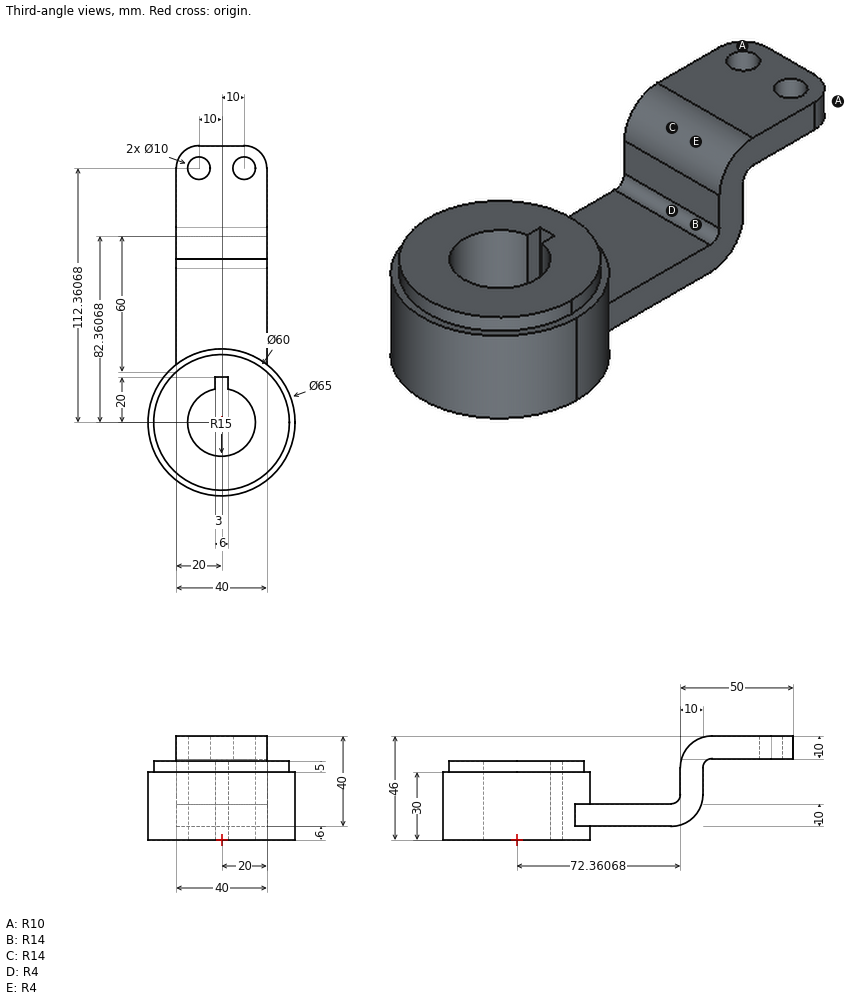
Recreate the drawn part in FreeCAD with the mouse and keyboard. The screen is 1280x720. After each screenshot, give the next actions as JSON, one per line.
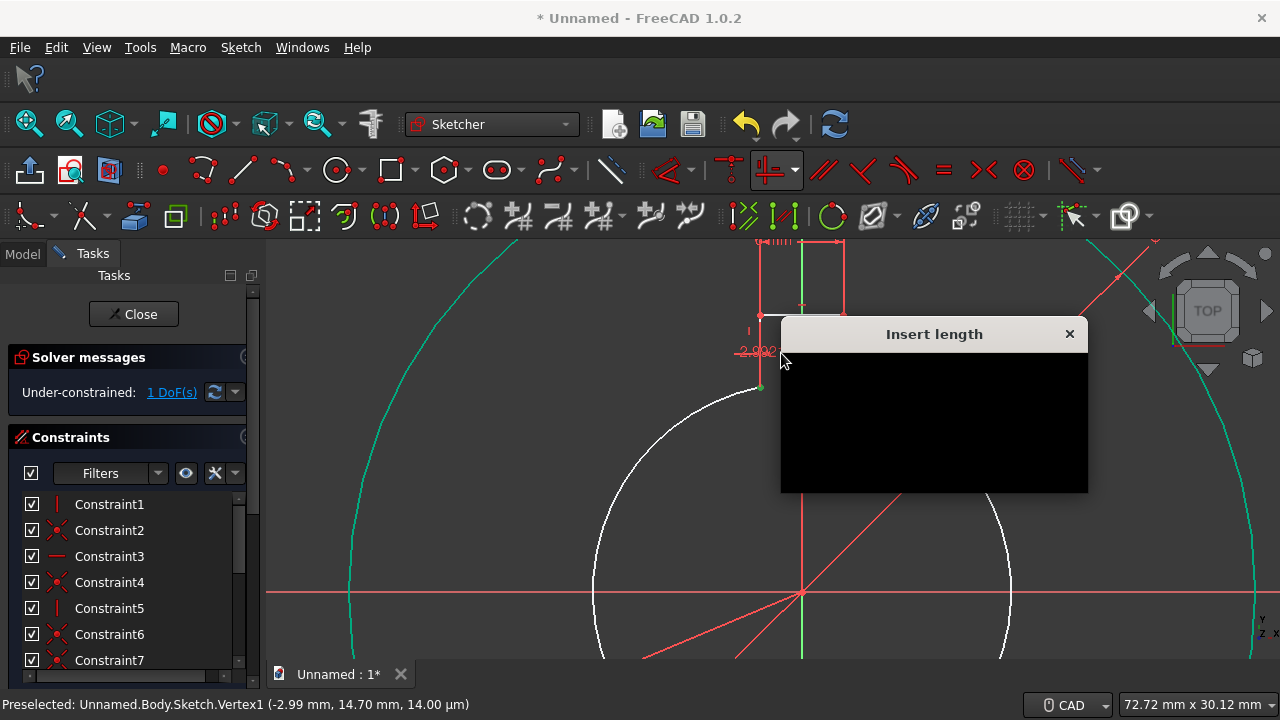
{"action": "type", "text": "3"}
{"action": "key", "text": "Return"}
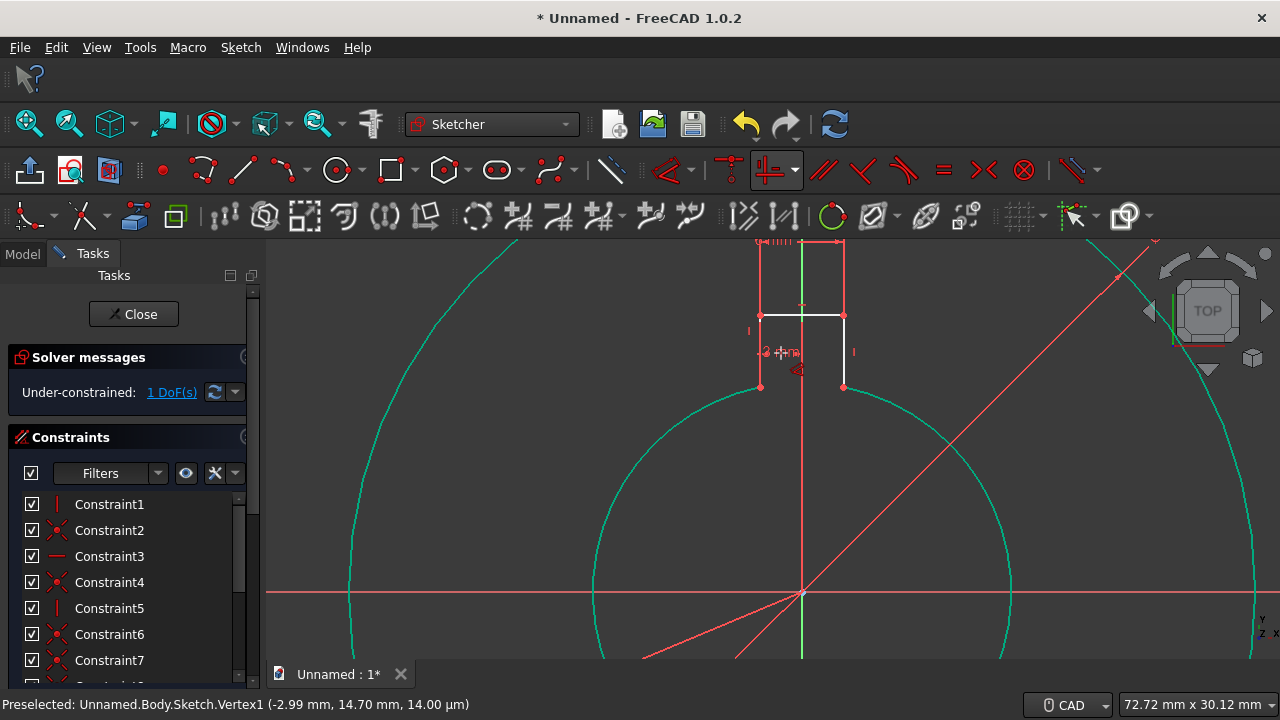
{"action": "left_click", "coordinate": [760, 315]}
{"action": "left_click", "coordinate": [726, 454]}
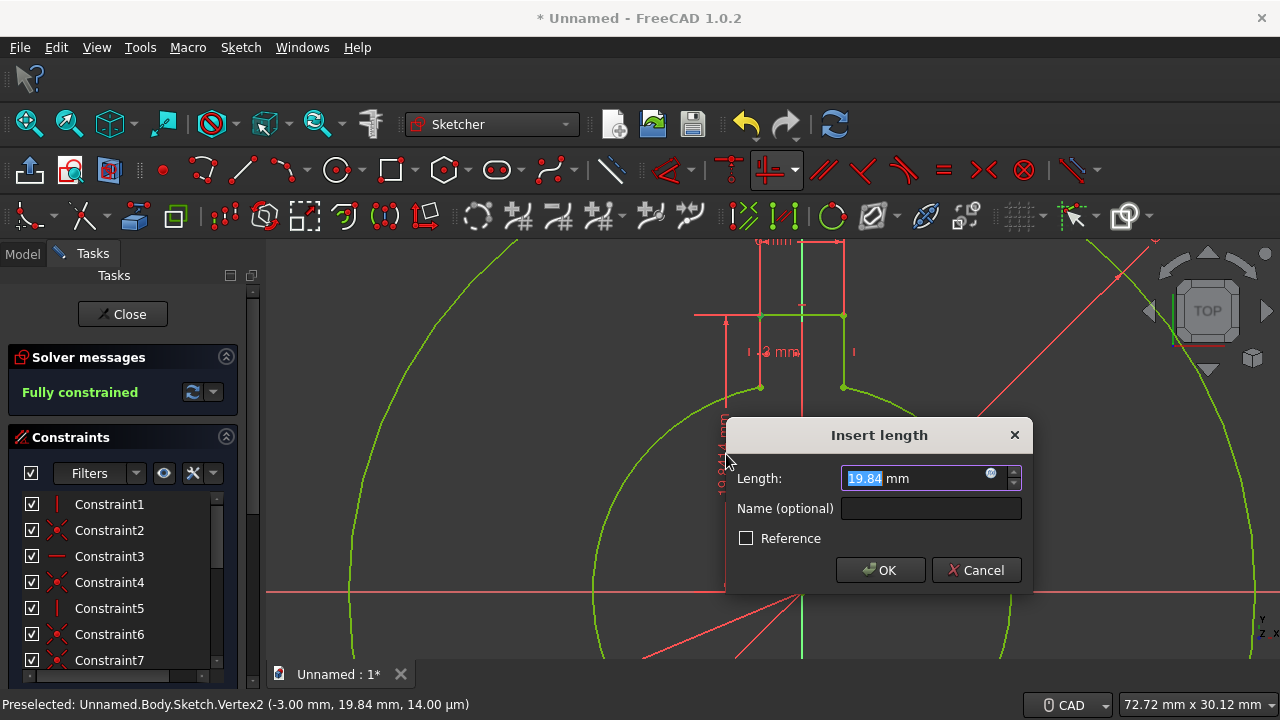
{"action": "type", "text": "20"}
{"action": "key", "text": "Return"}
{"action": "key", "text": "Escape"}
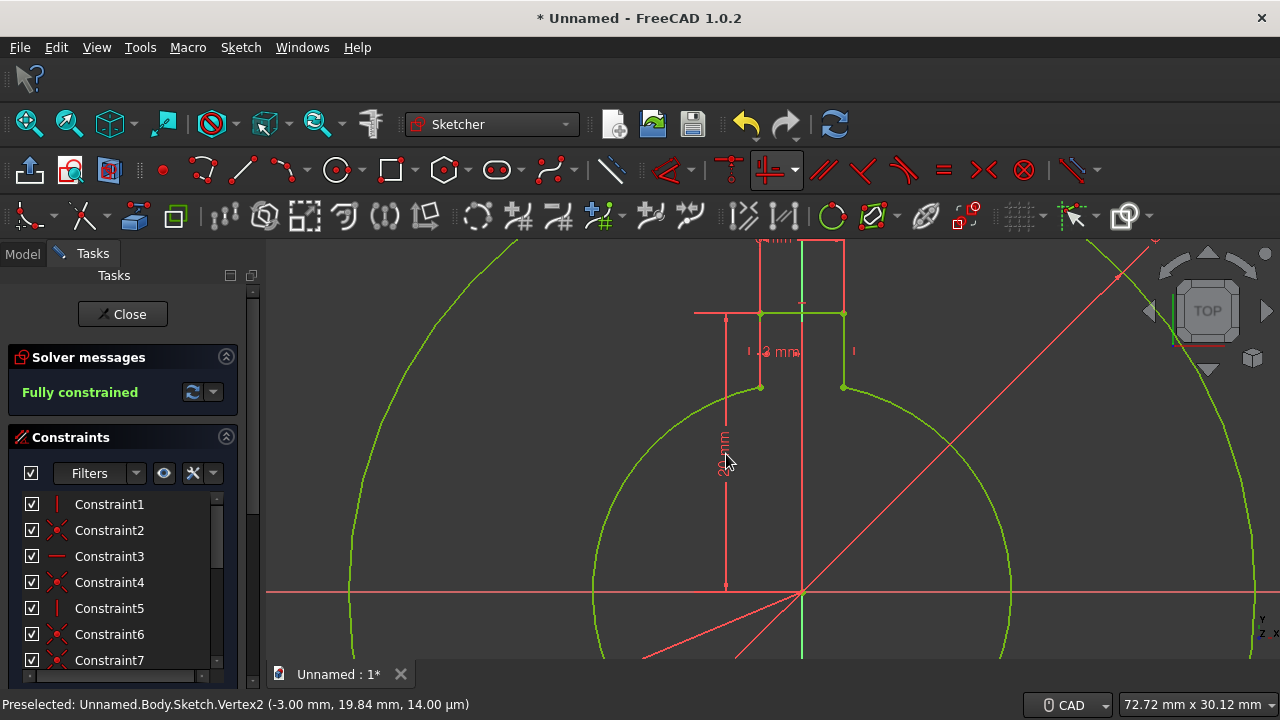
{"action": "left_click", "coordinate": [123, 314]}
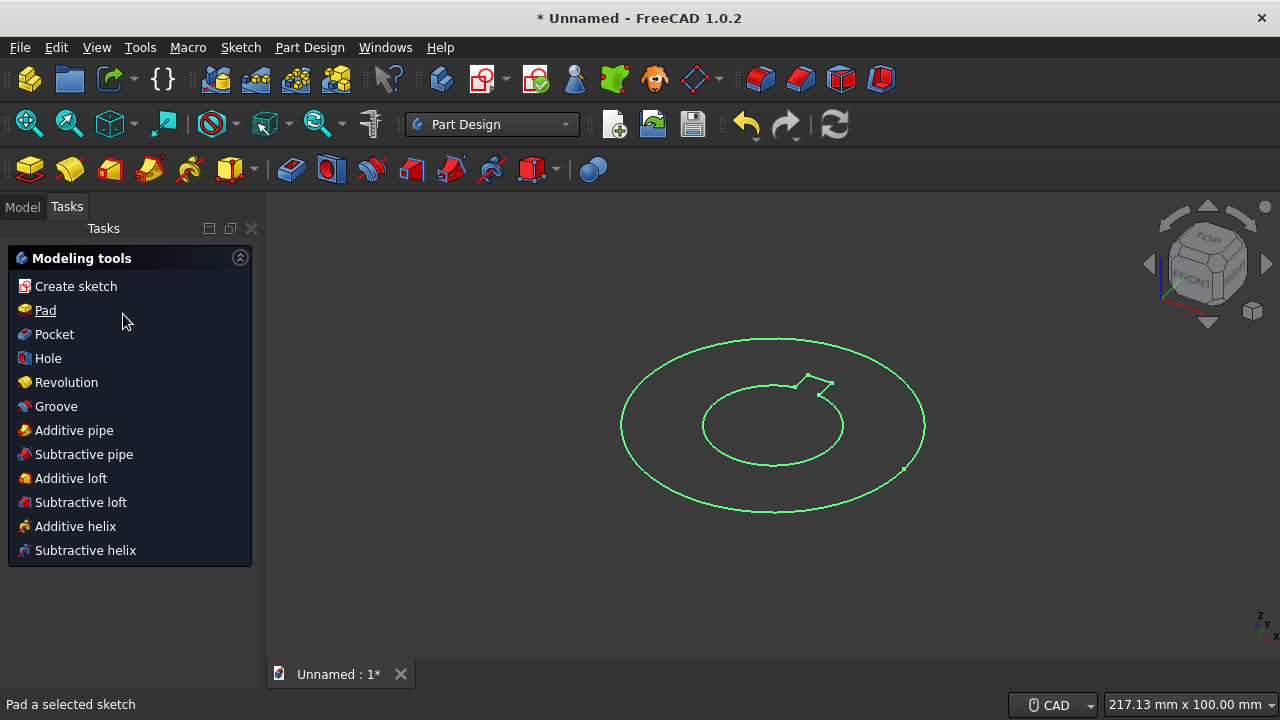
{"action": "left_click", "coordinate": [30, 170]}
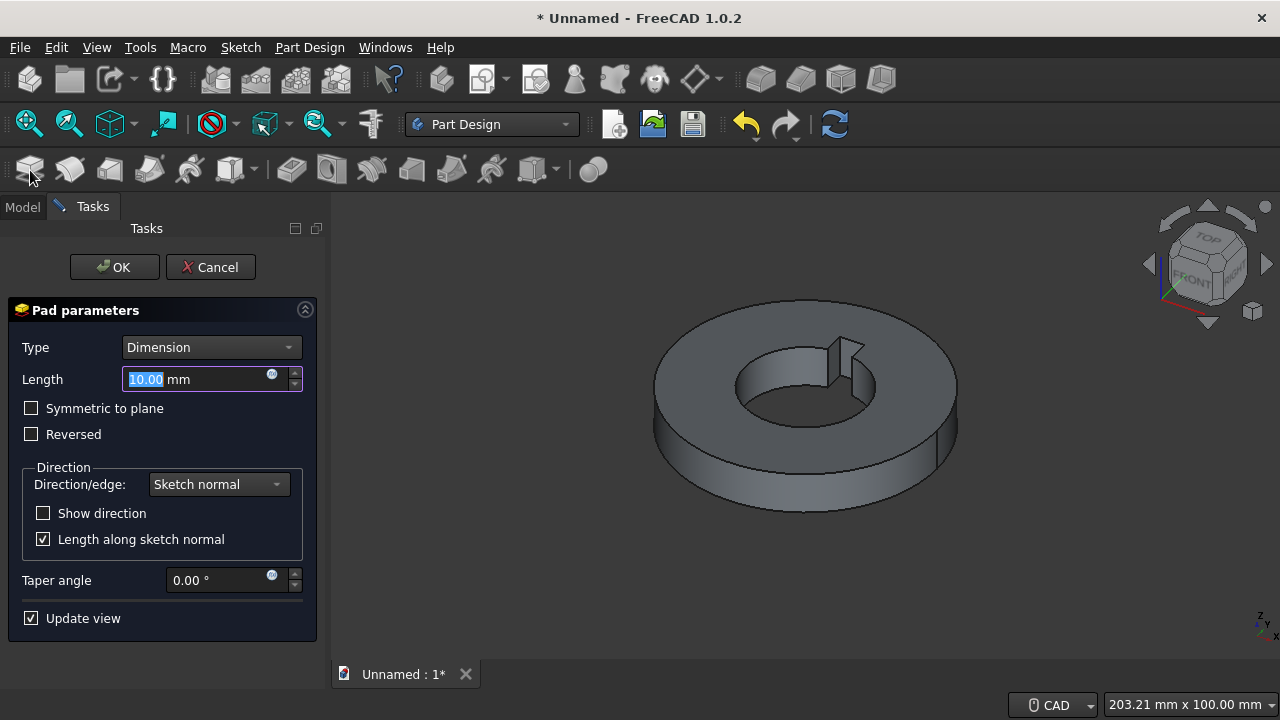
{"action": "type", "text": "30"}
{"action": "key", "text": "Tab"}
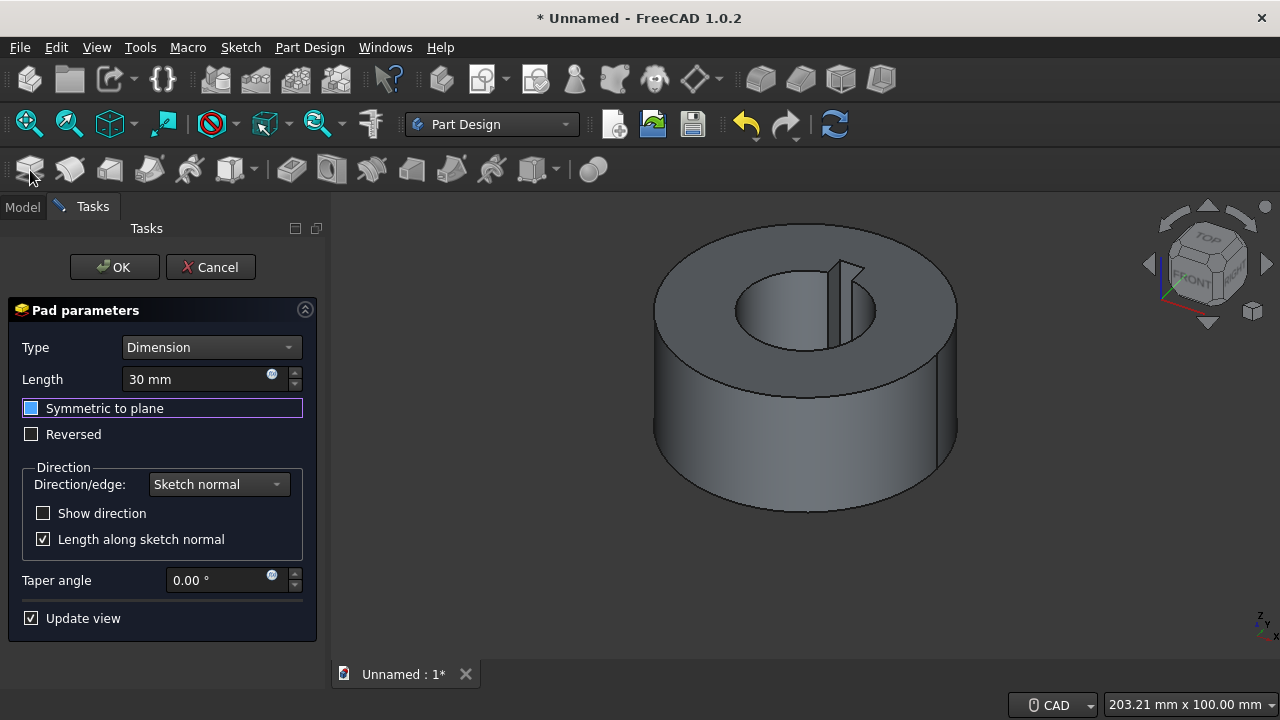
{"action": "left_click", "coordinate": [115, 267]}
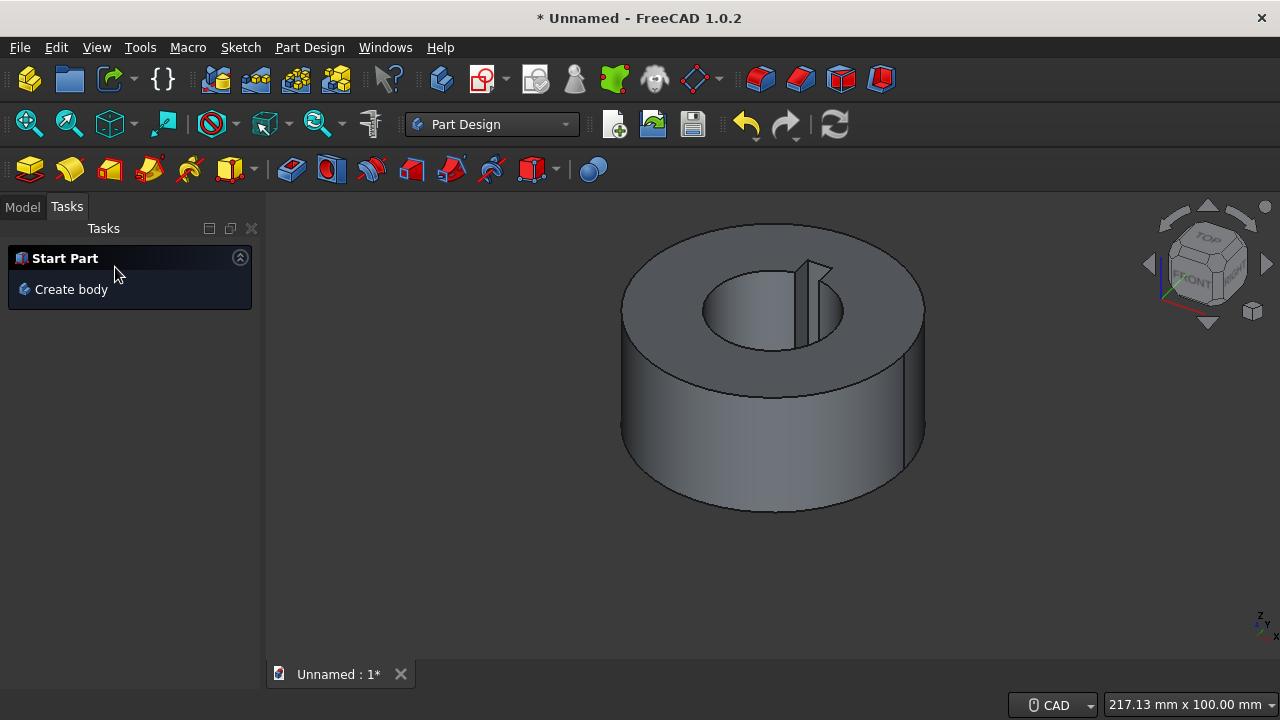
{"action": "key", "text": "v f"}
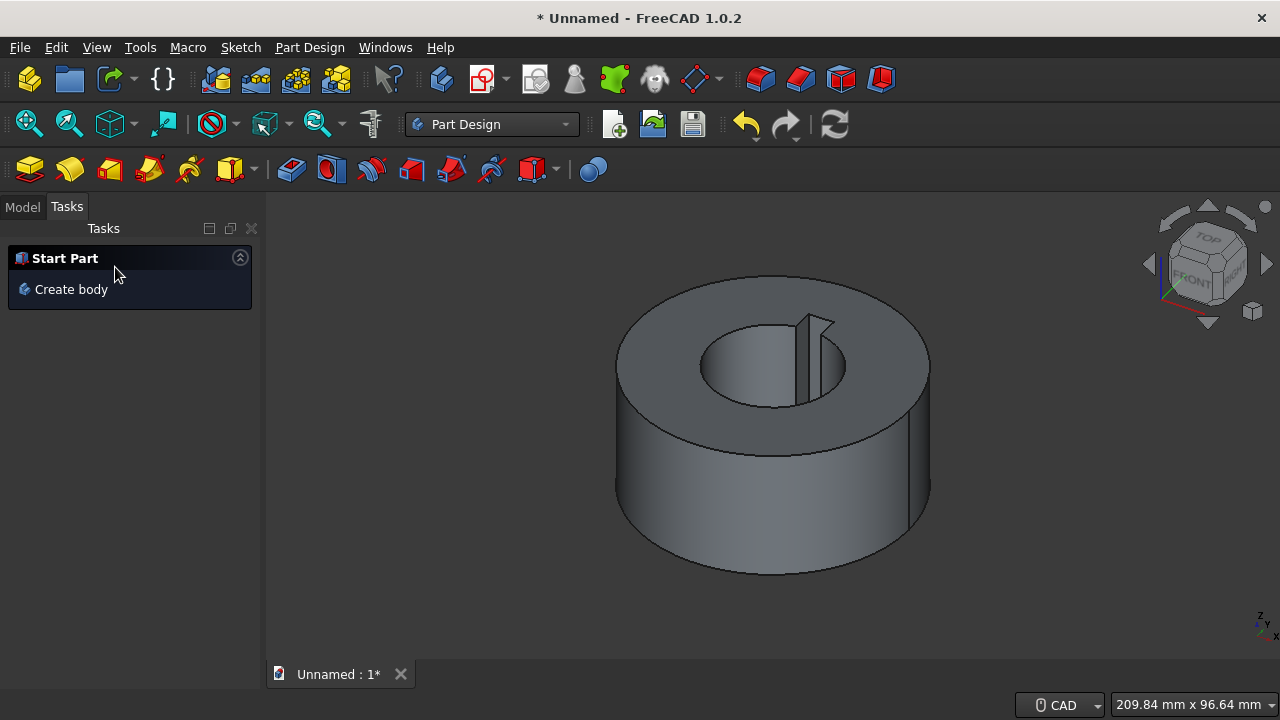
{"action": "left_click", "coordinate": [650, 384]}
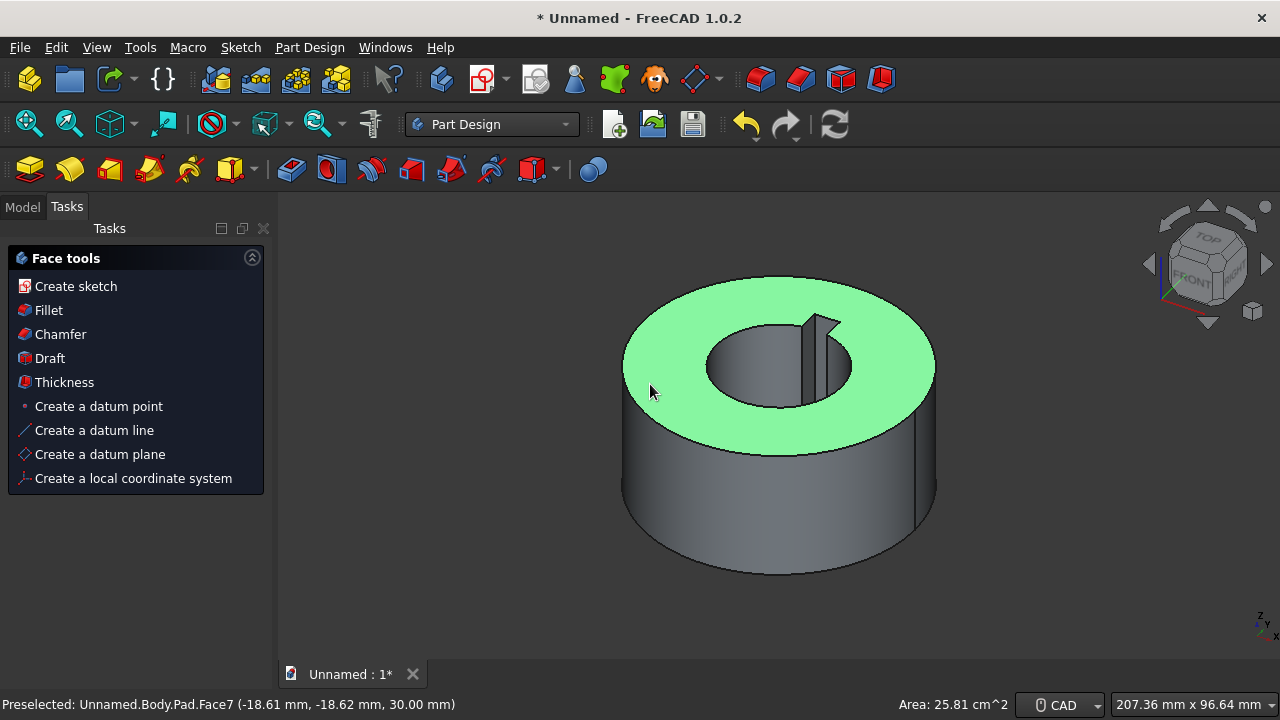
{"action": "left_click", "coordinate": [482, 80]}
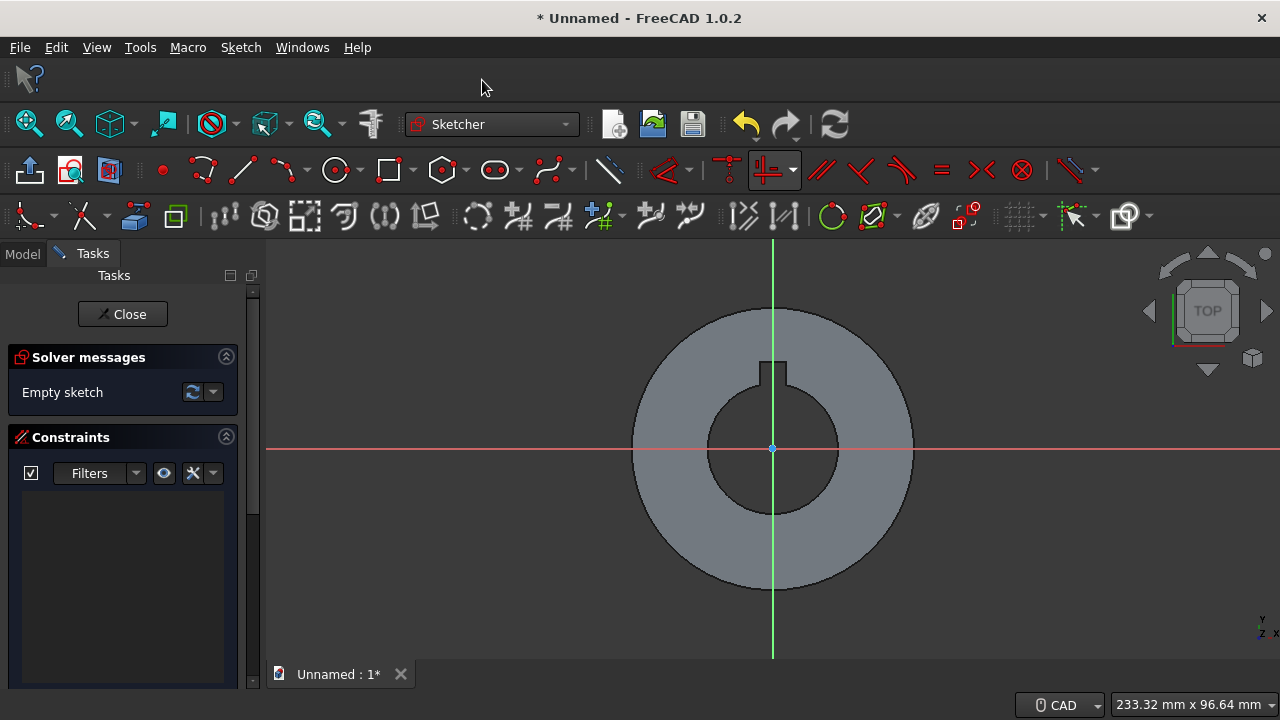
{"action": "left_click", "coordinate": [204, 170]}